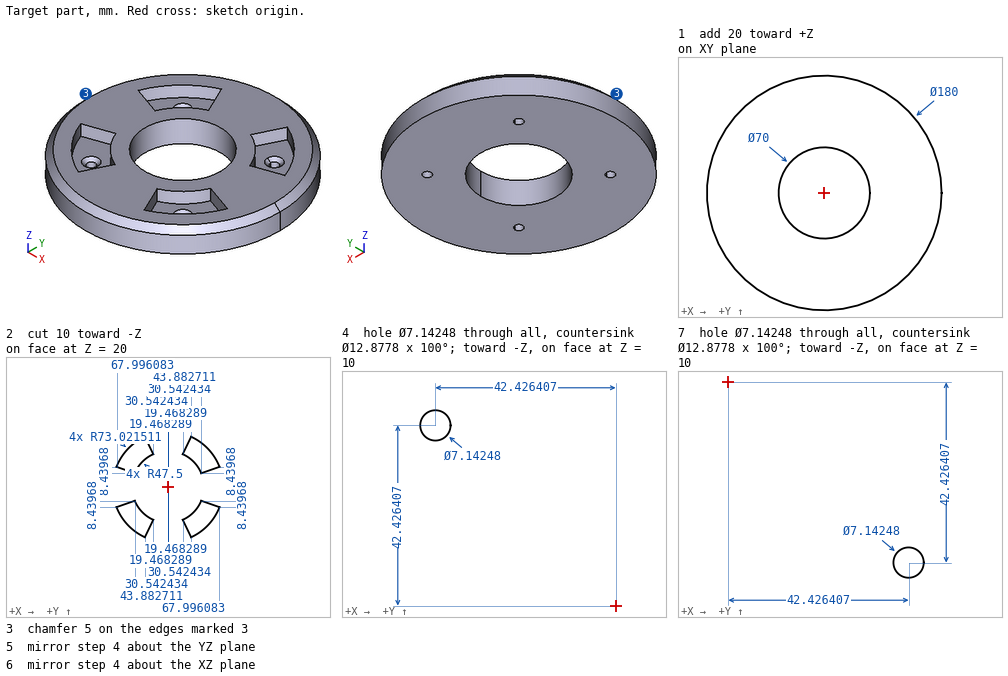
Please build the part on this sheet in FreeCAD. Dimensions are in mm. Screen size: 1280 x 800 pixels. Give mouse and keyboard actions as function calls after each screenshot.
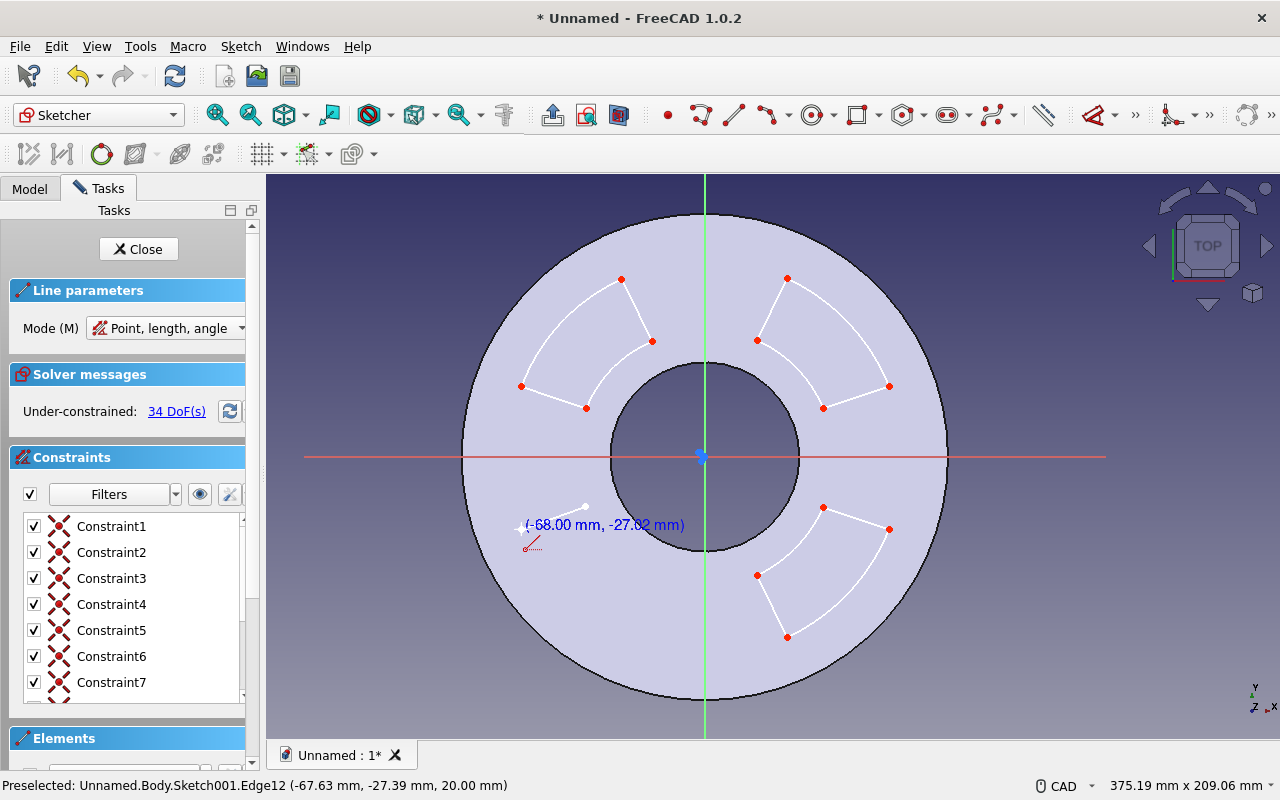
click(622, 636)
click(652, 574)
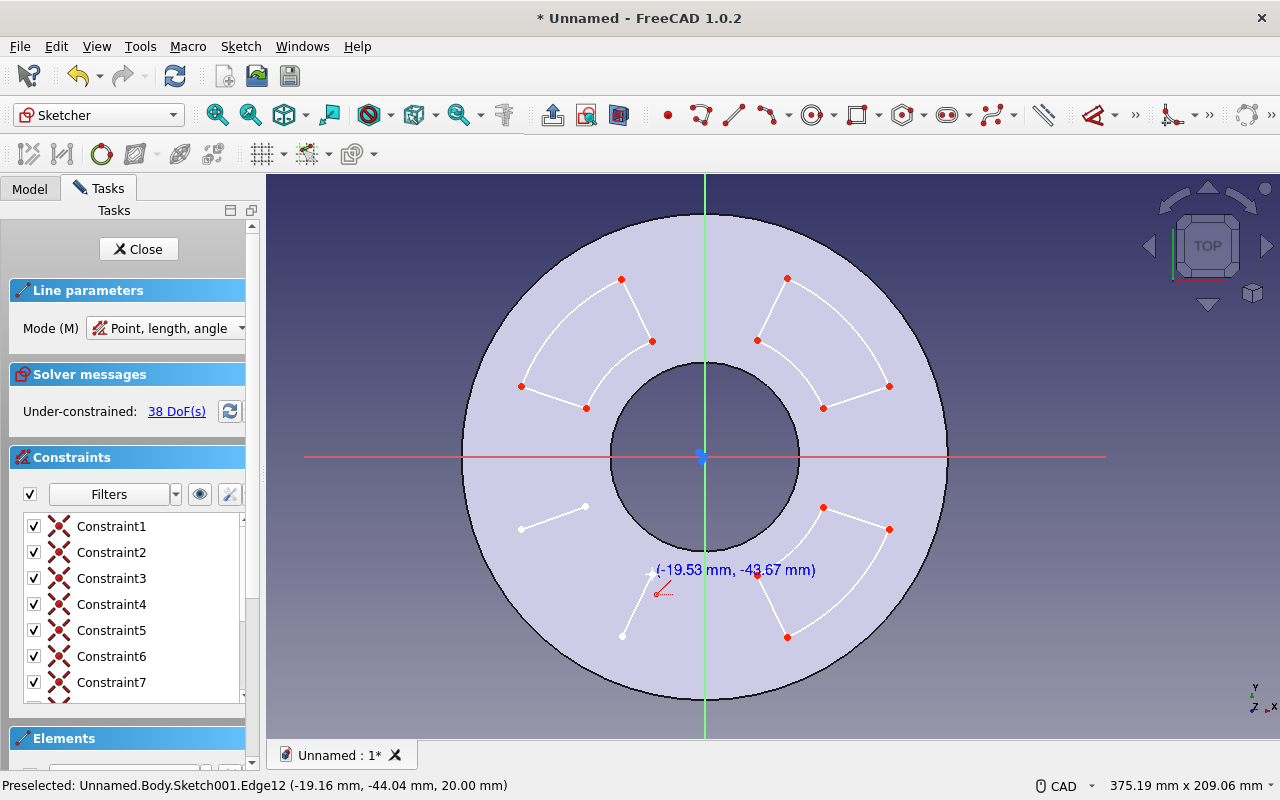
click(766, 116)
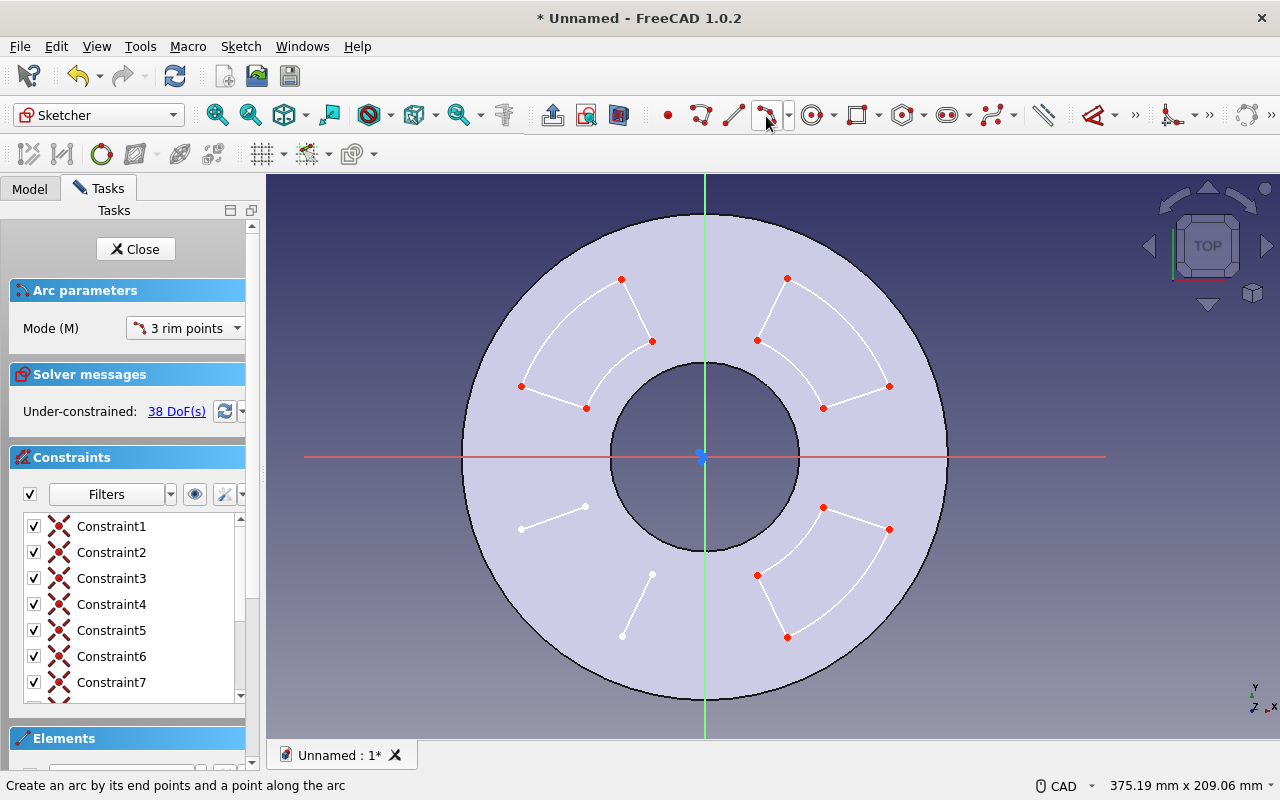
click(521, 530)
click(622, 637)
click(561, 592)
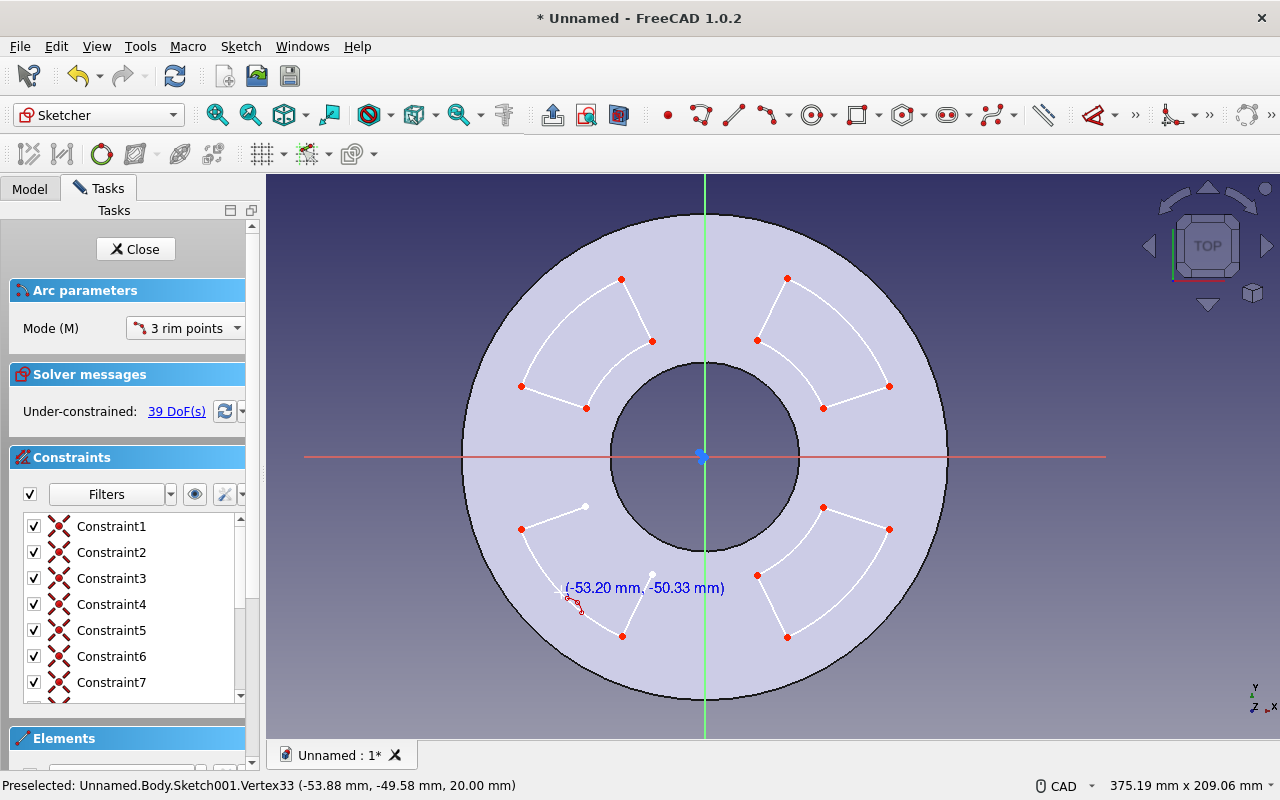
click(652, 575)
click(586, 507)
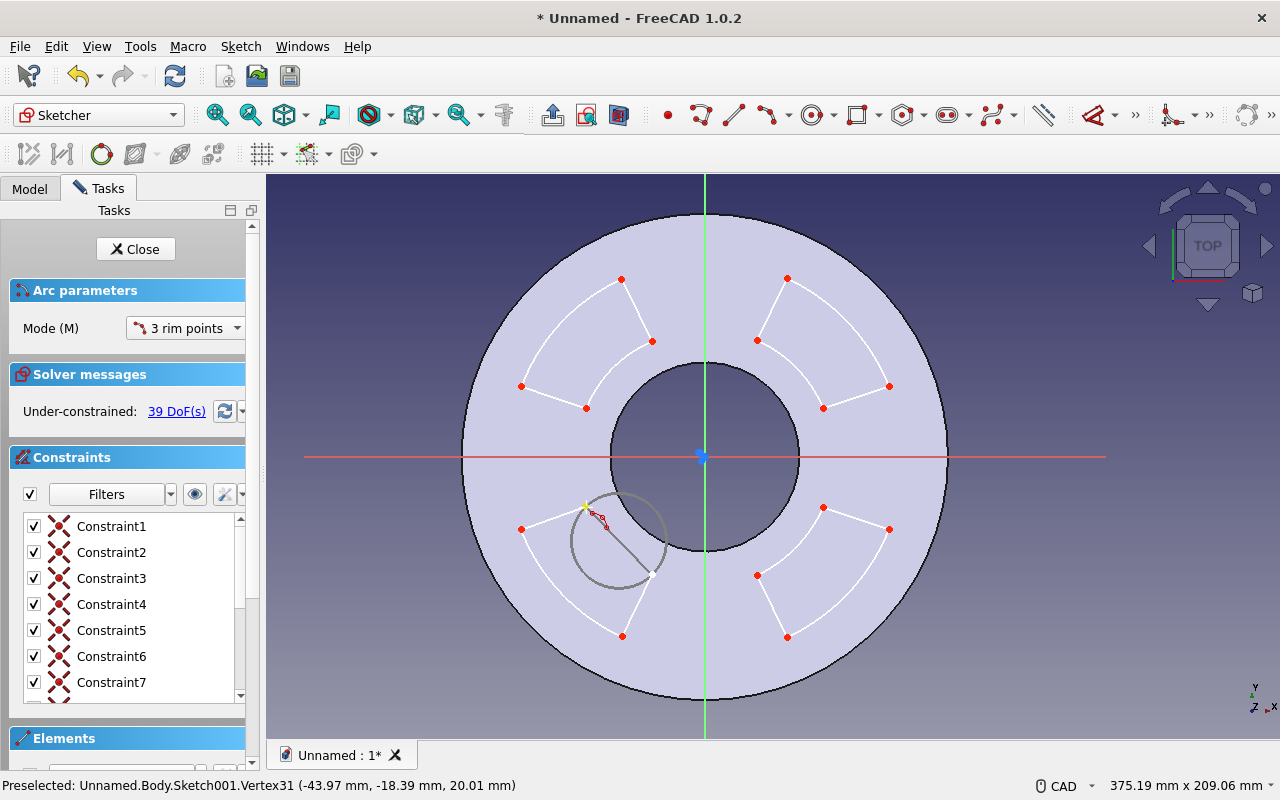
scroll(613, 546, up, 3)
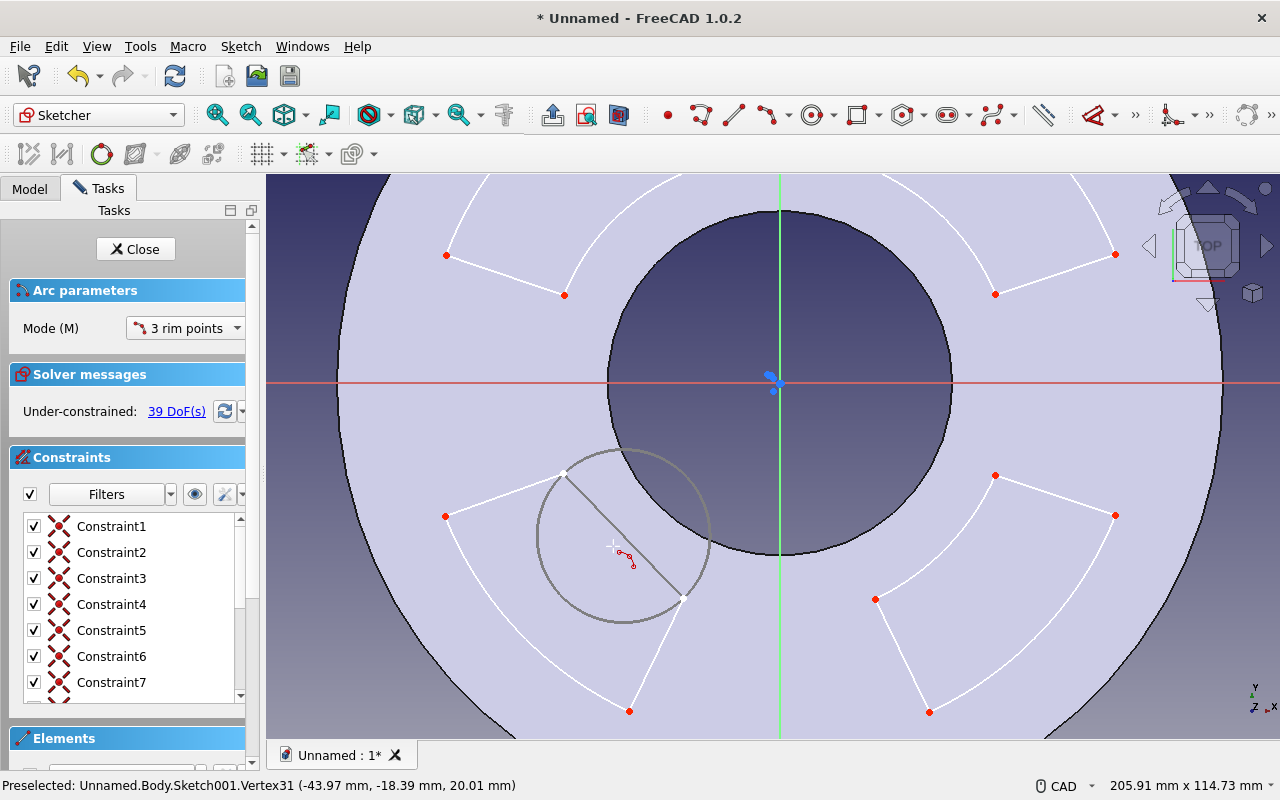
click(612, 546)
key(Escape)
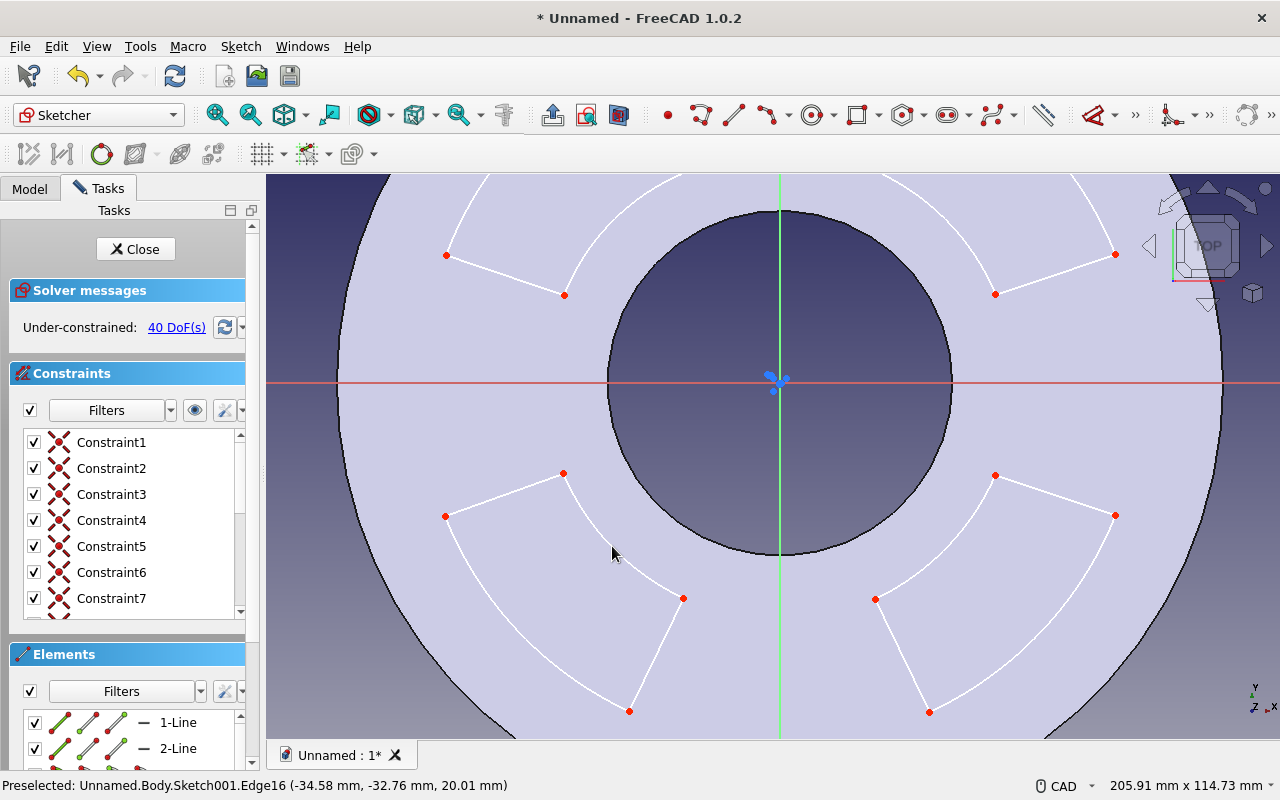
click(469, 205)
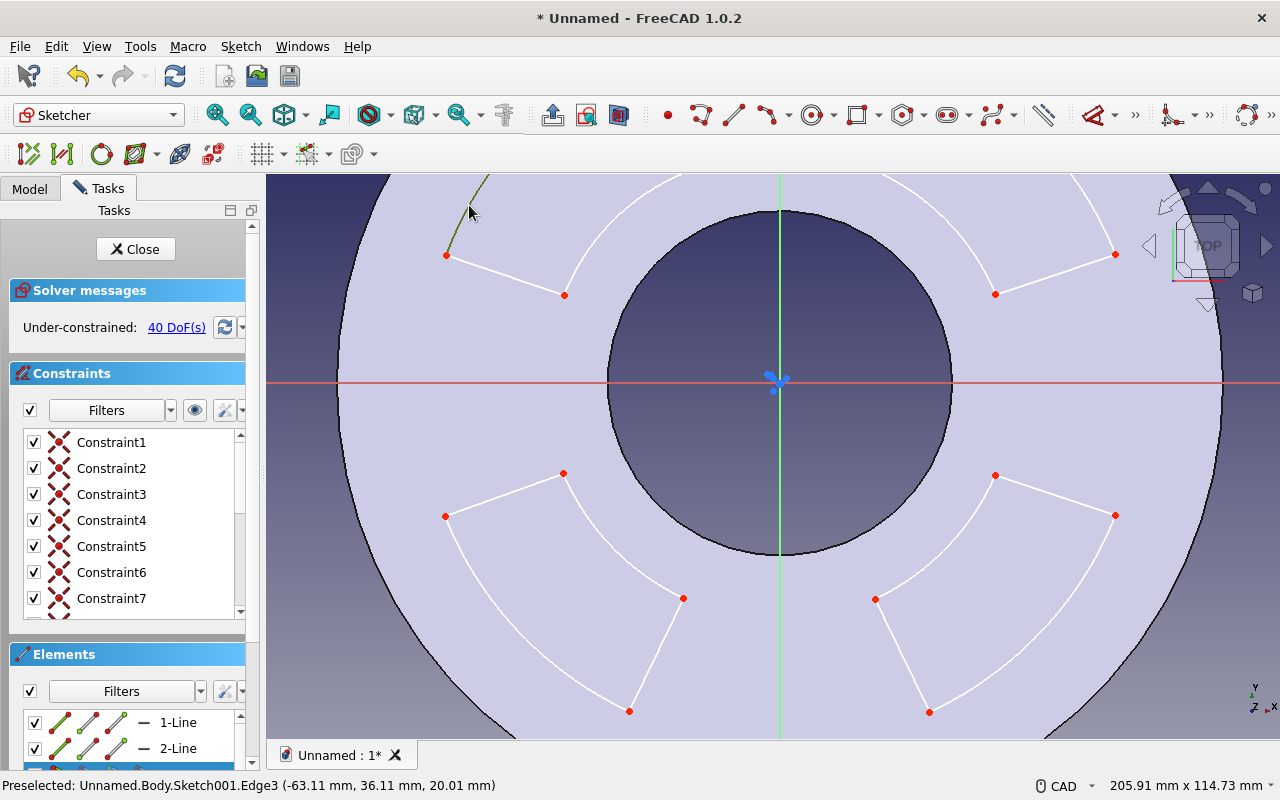
click(589, 249)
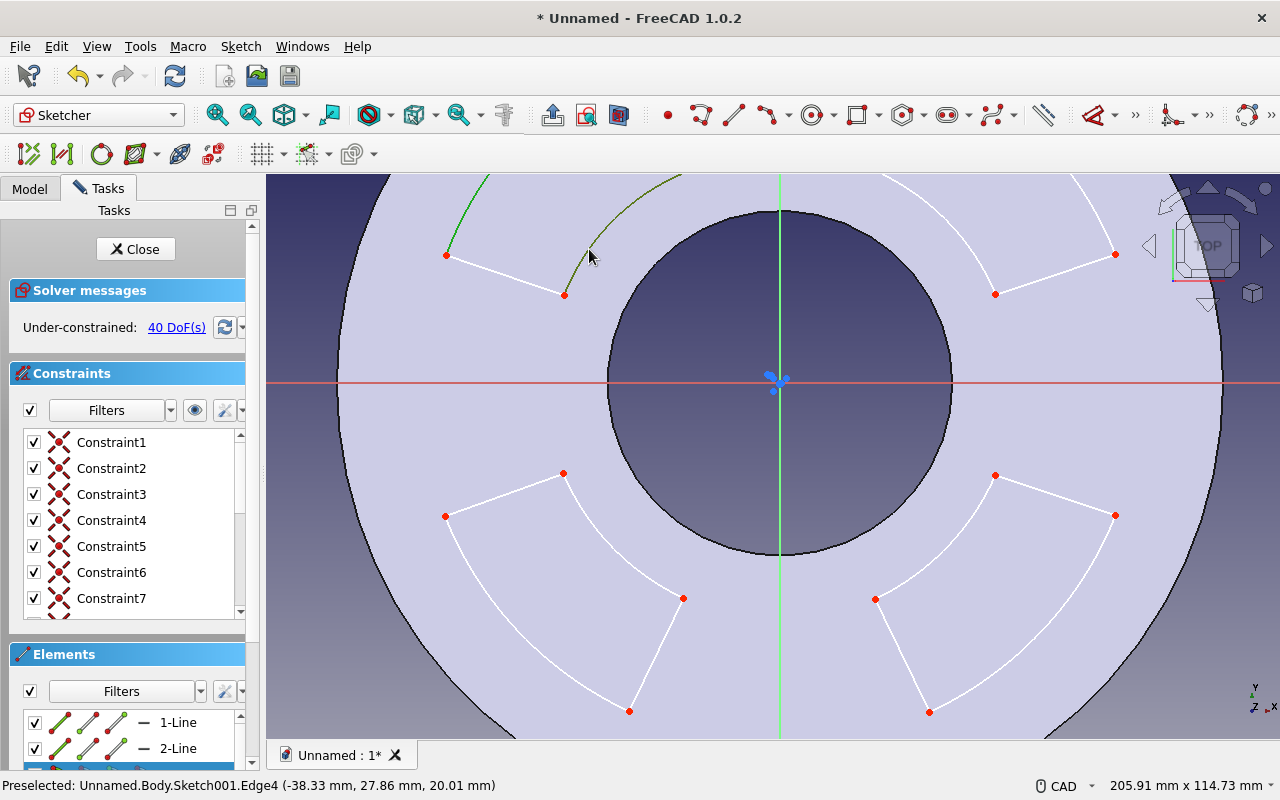
key(c)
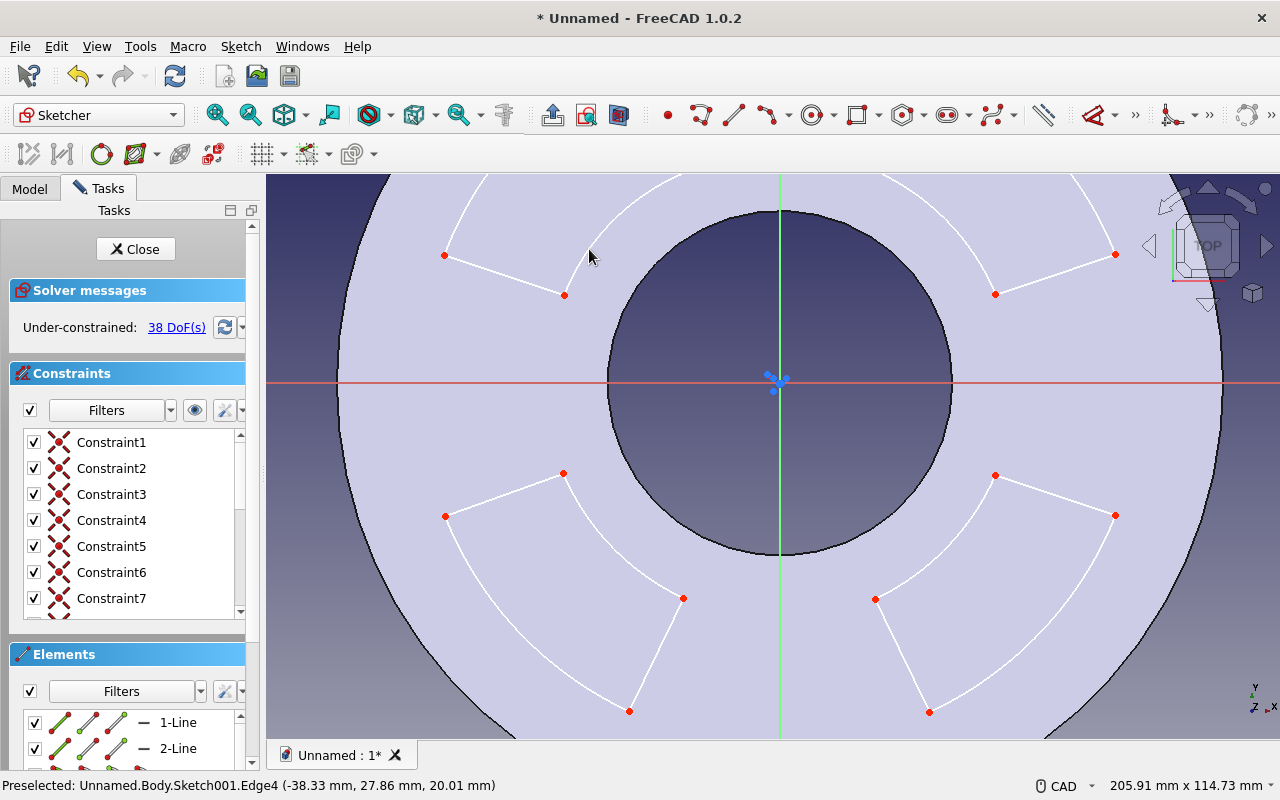
click(468, 205)